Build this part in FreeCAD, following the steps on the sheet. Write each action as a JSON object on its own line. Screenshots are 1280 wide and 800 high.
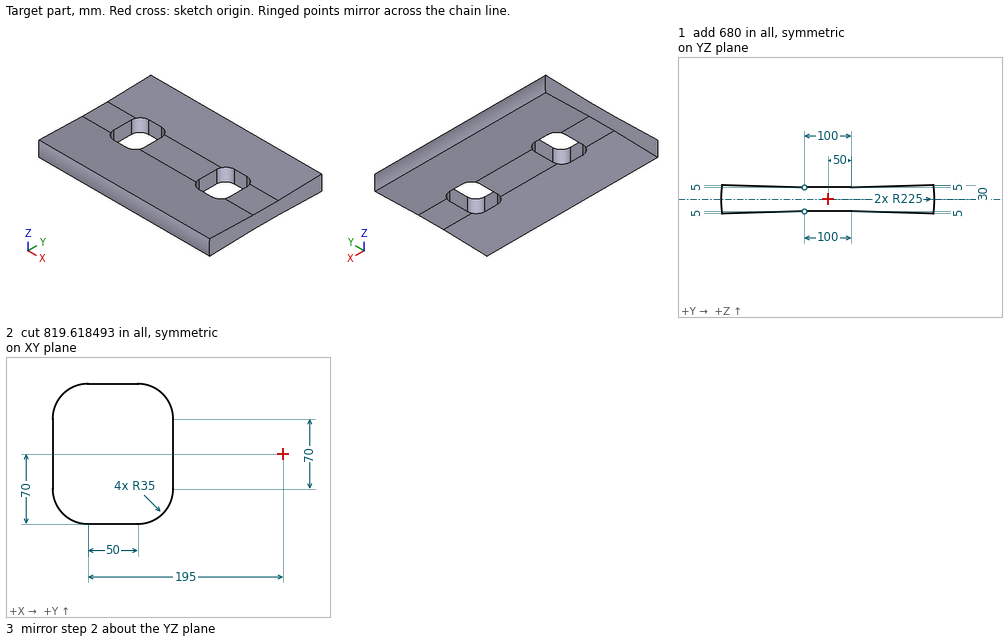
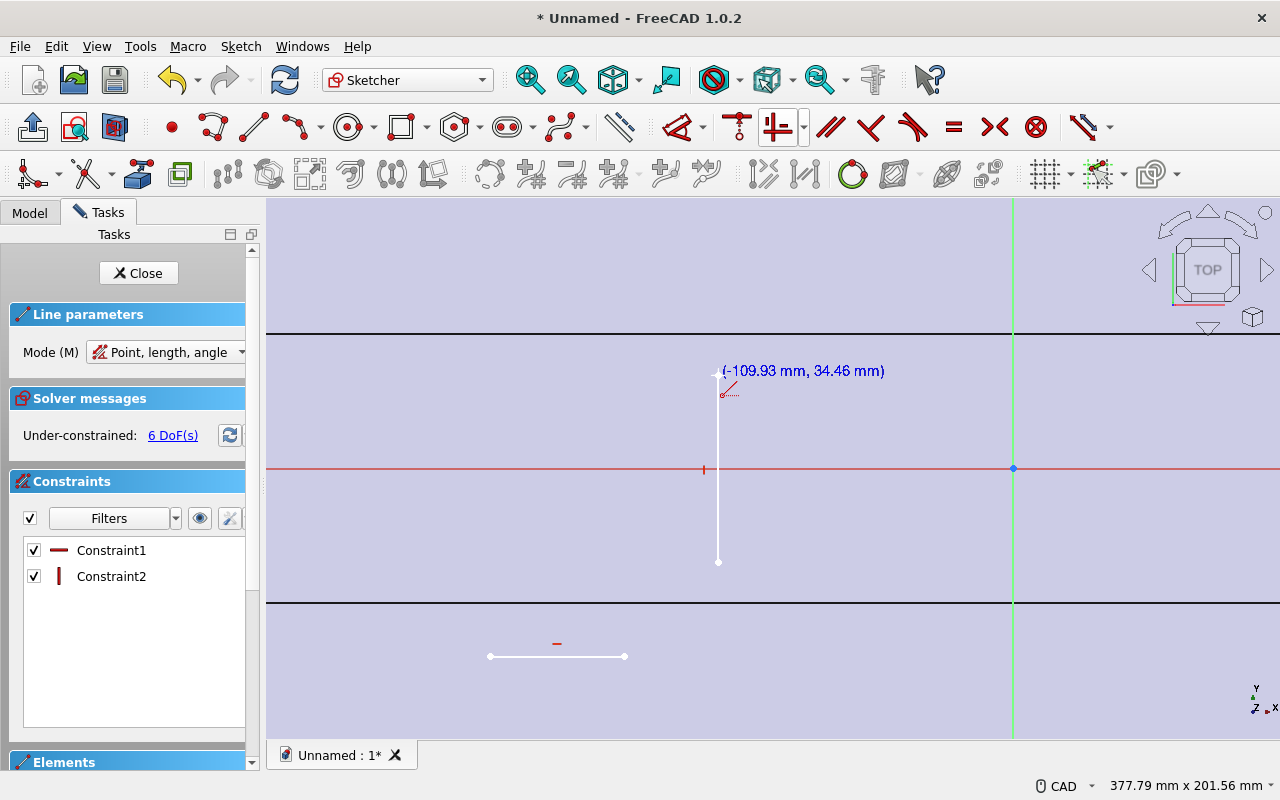
{"action": "left_click", "coordinate": [624, 281]}
{"action": "left_click", "coordinate": [490, 281]}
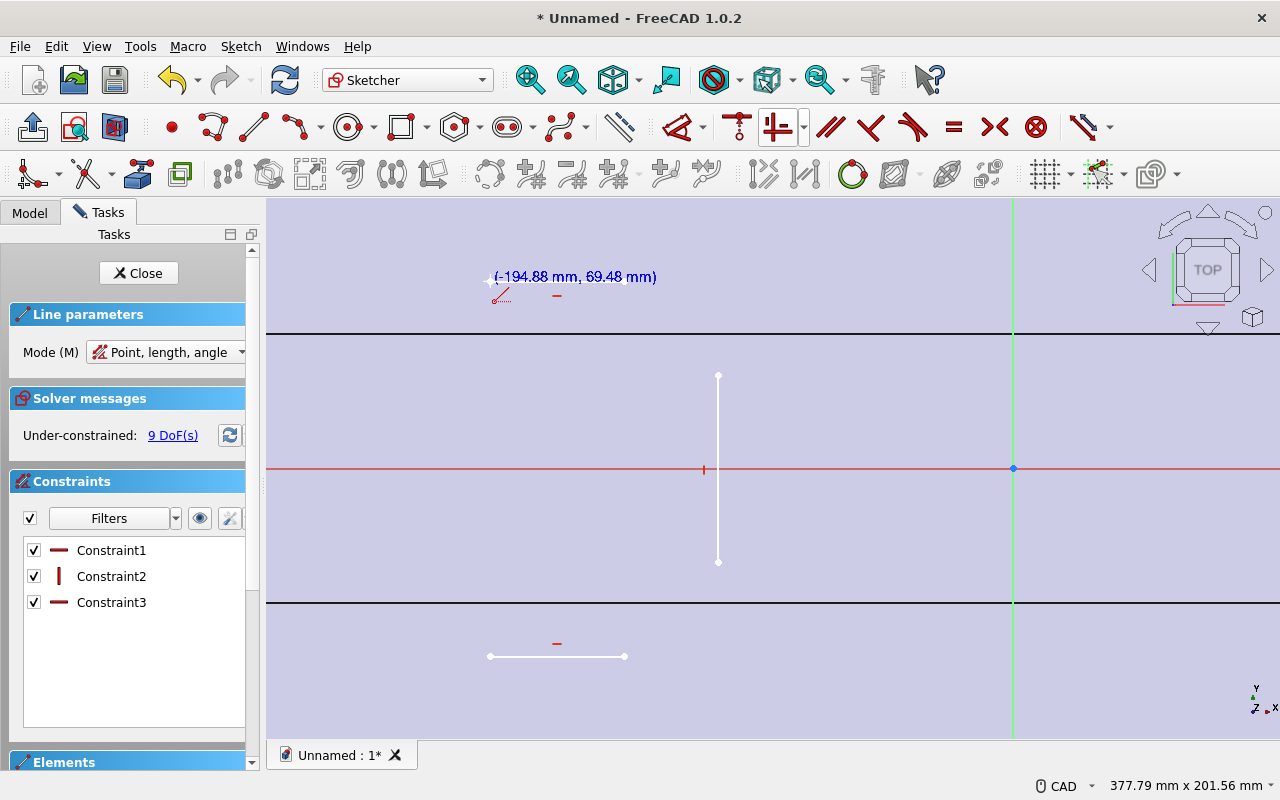
{"action": "left_click", "coordinate": [396, 375]}
{"action": "left_click", "coordinate": [396, 562]}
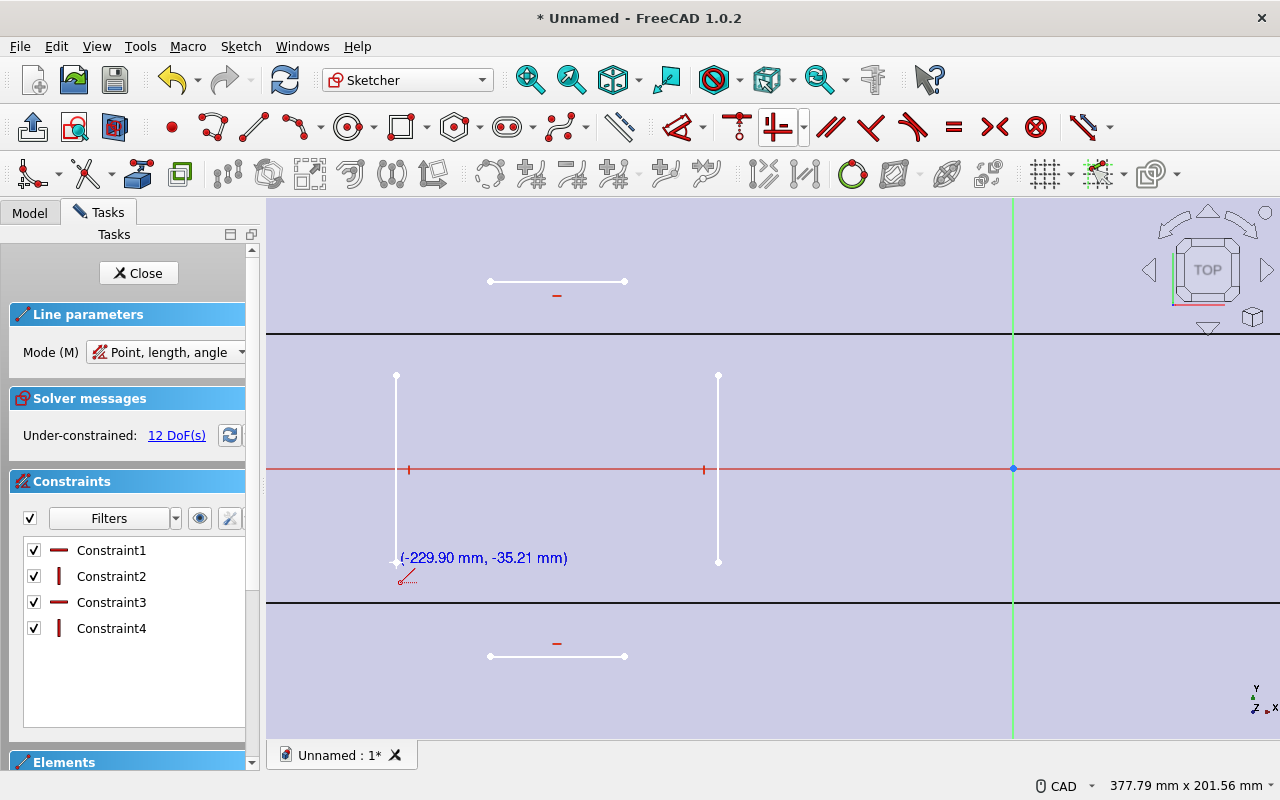
{"action": "key", "text": "g 3 a"}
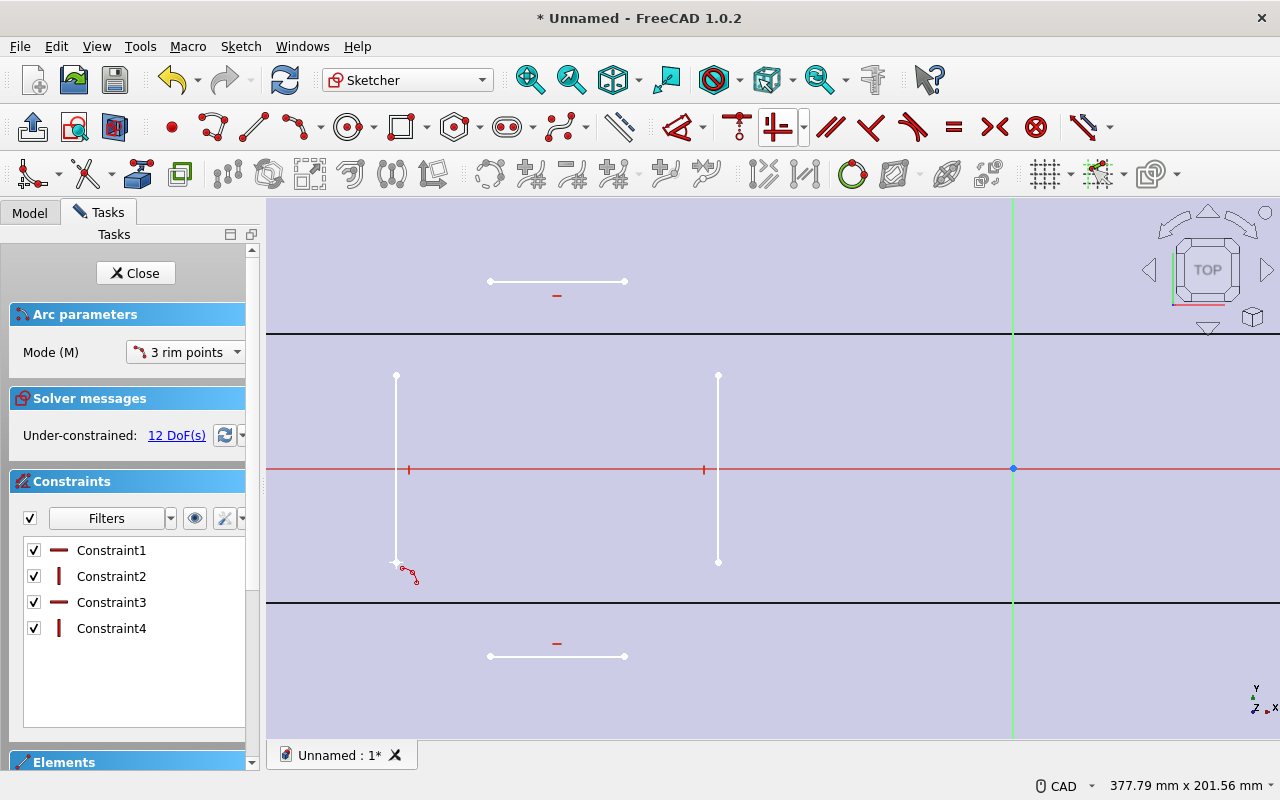
{"action": "left_click", "coordinate": [624, 657]}
{"action": "left_click", "coordinate": [718, 563]}
{"action": "left_click", "coordinate": [690, 629]}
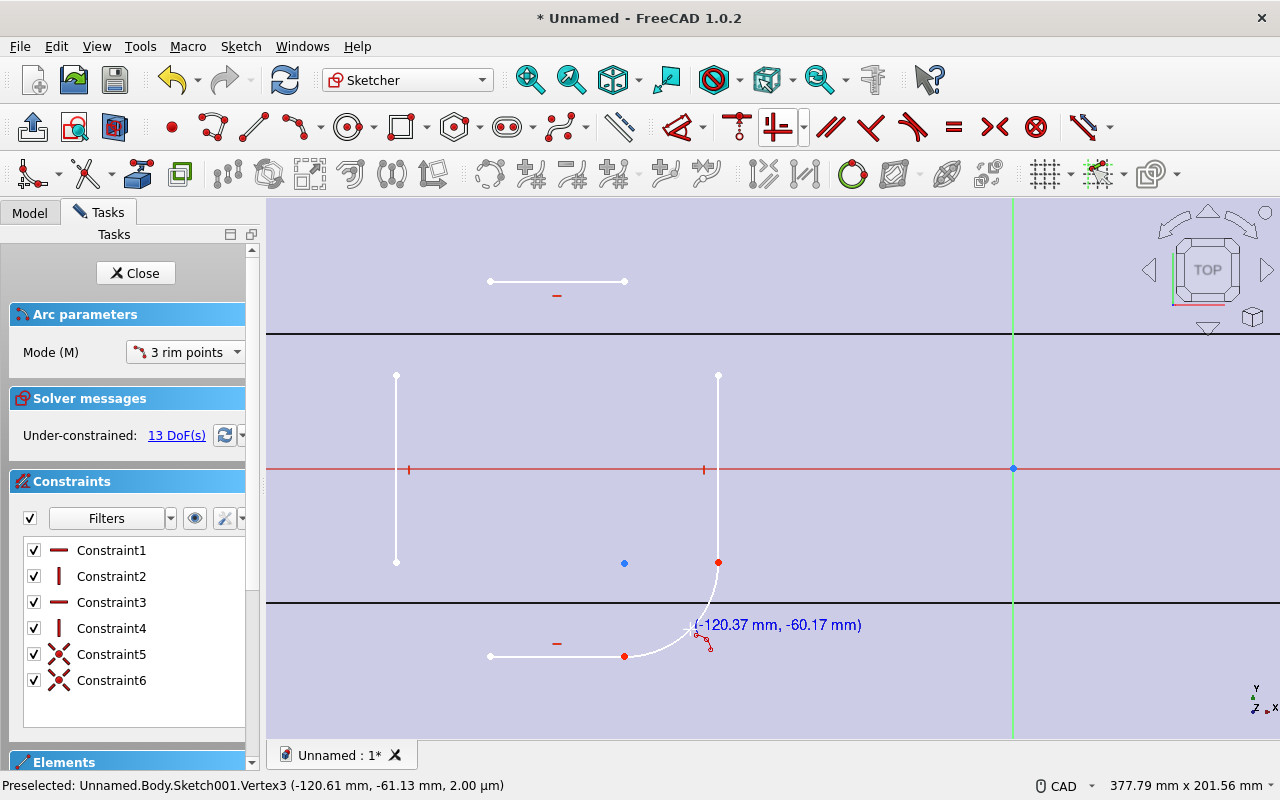
{"action": "left_click", "coordinate": [718, 376]}
{"action": "left_click", "coordinate": [624, 282]}
{"action": "left_click", "coordinate": [690, 308]}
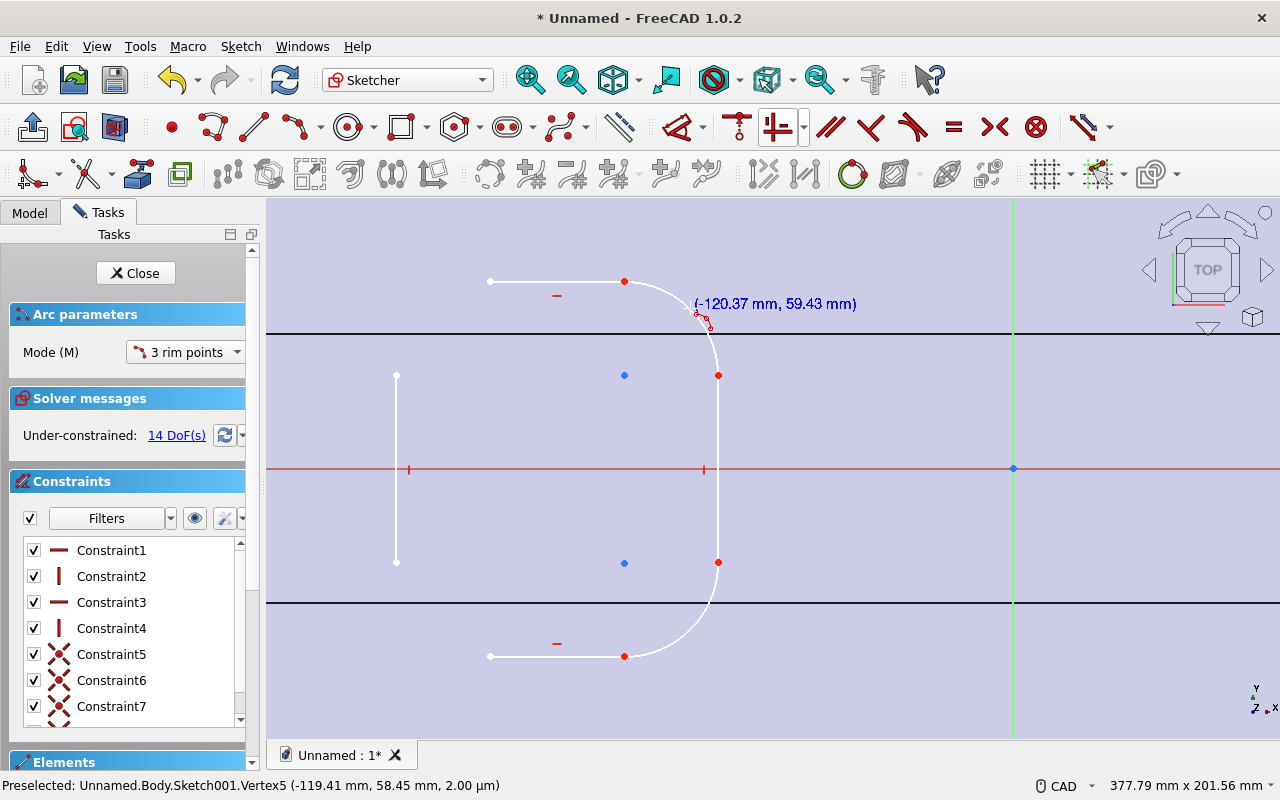
{"action": "left_click", "coordinate": [490, 282]}
{"action": "left_click", "coordinate": [396, 376]}
{"action": "left_click", "coordinate": [423, 308]}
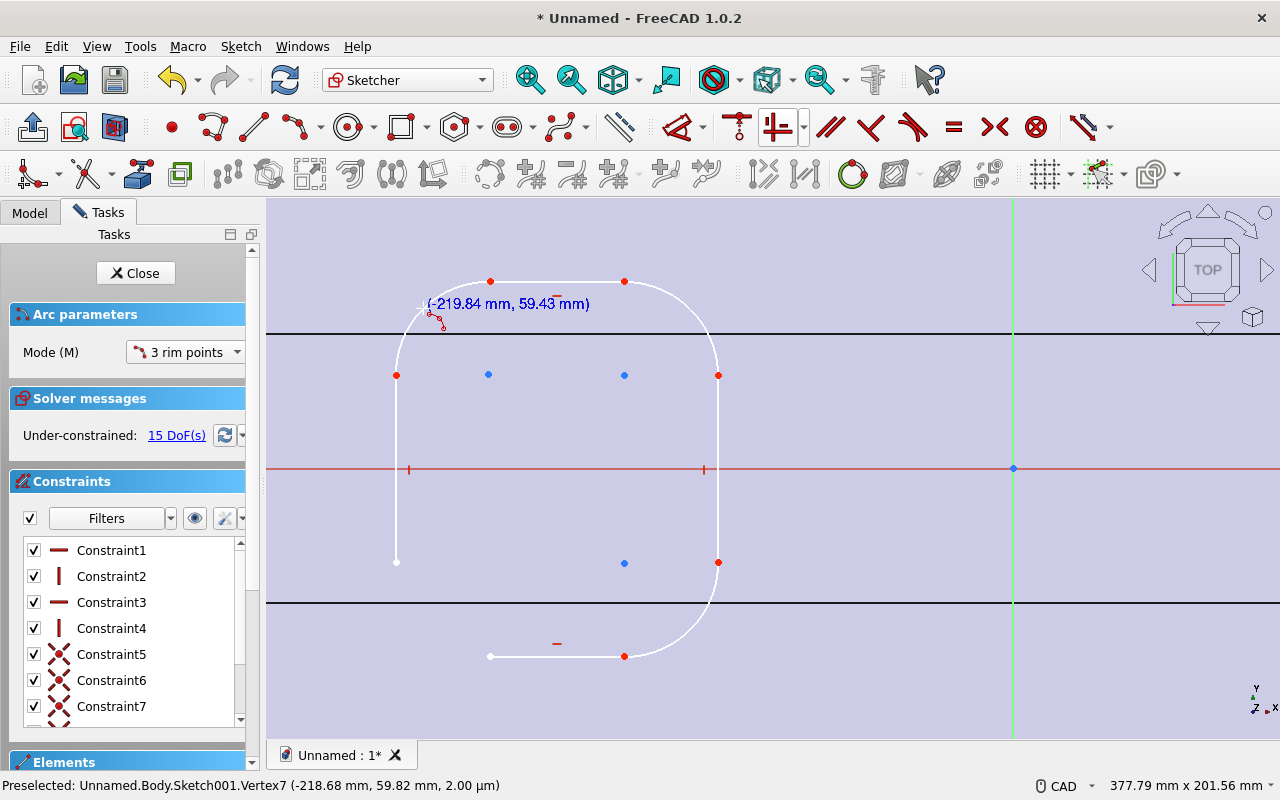
{"action": "left_click", "coordinate": [396, 563]}
{"action": "left_click", "coordinate": [490, 657]}
{"action": "left_click", "coordinate": [423, 629]}
{"action": "key", "text": "Escape"}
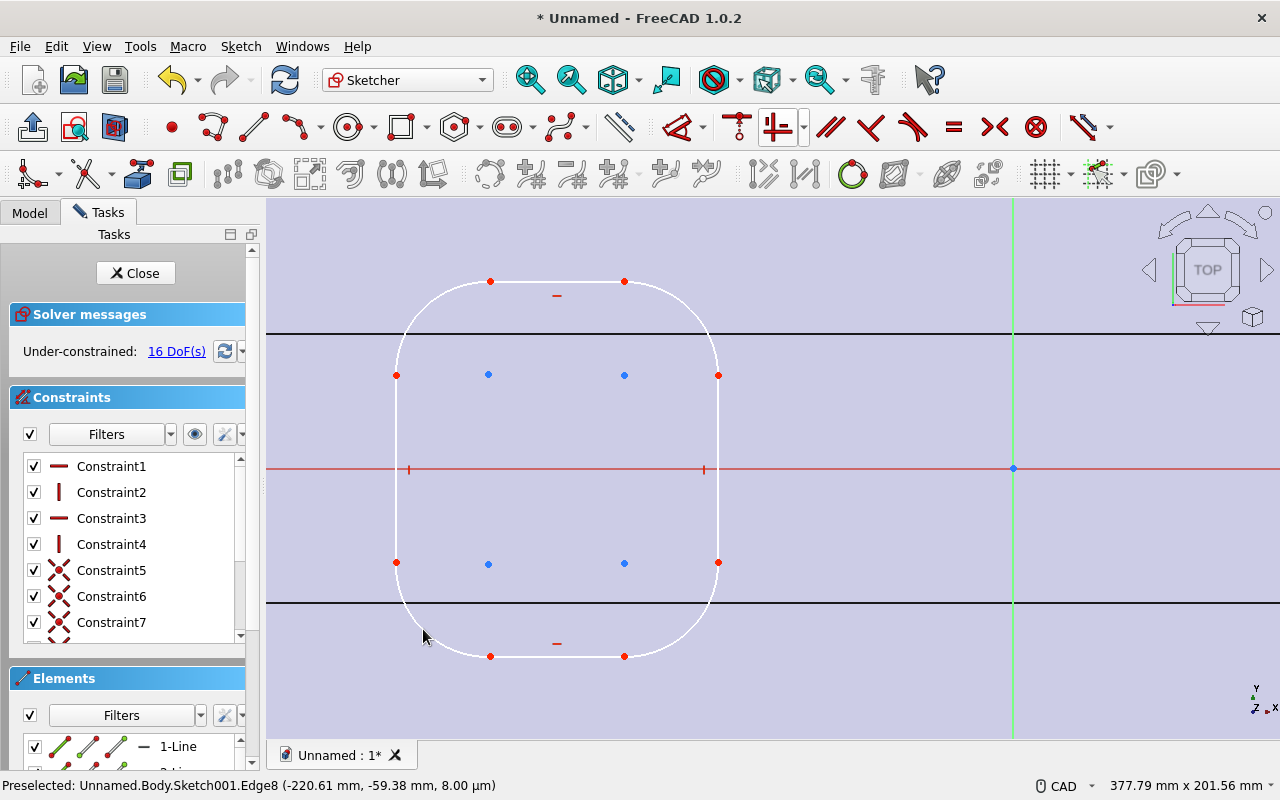
{"action": "left_click", "coordinate": [530, 657]}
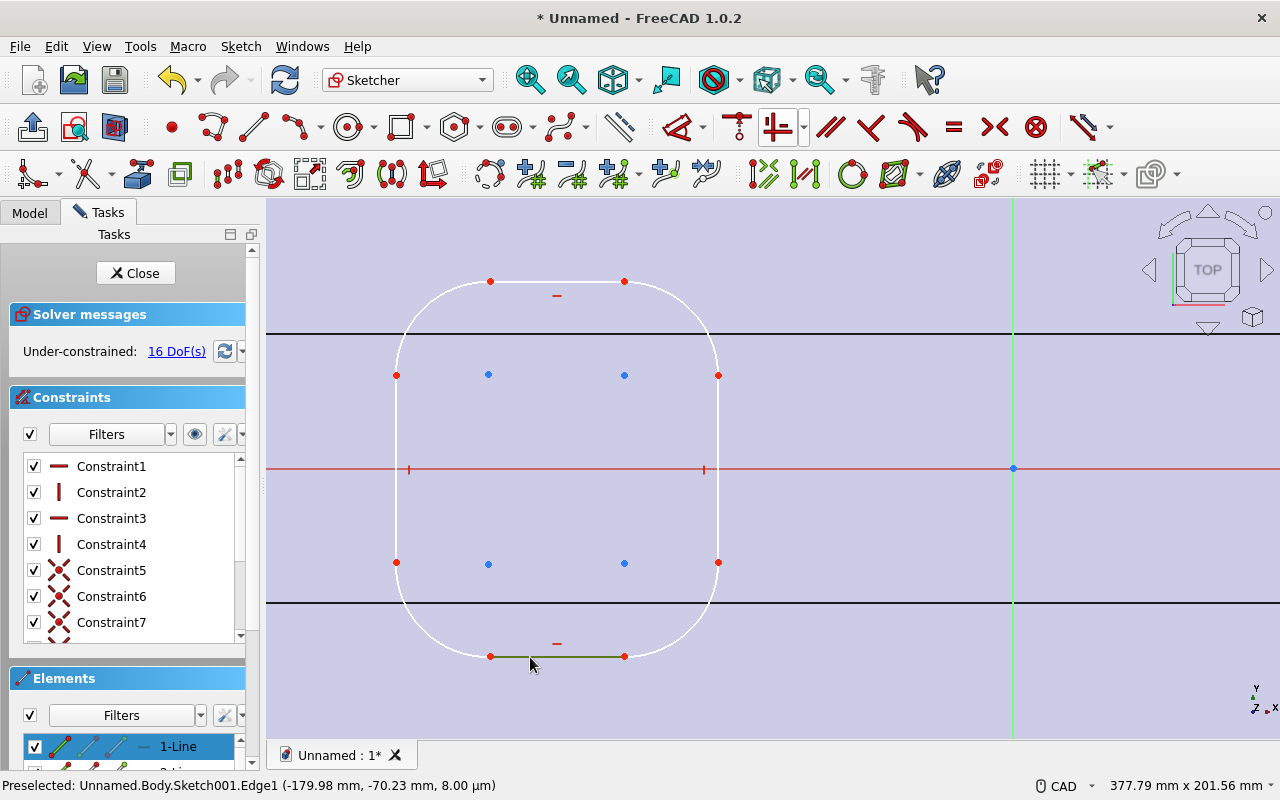
{"action": "left_click", "coordinate": [667, 647]}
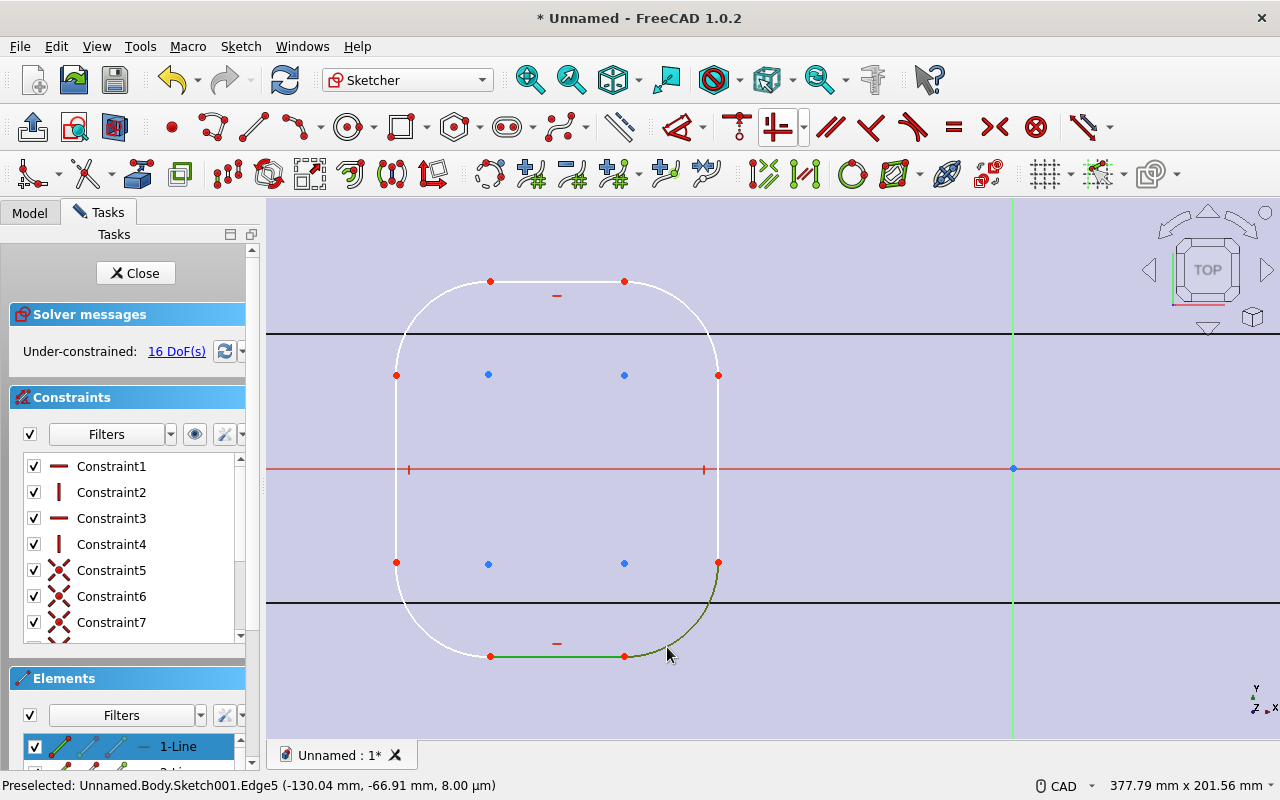
{"action": "left_click", "coordinate": [913, 128]}